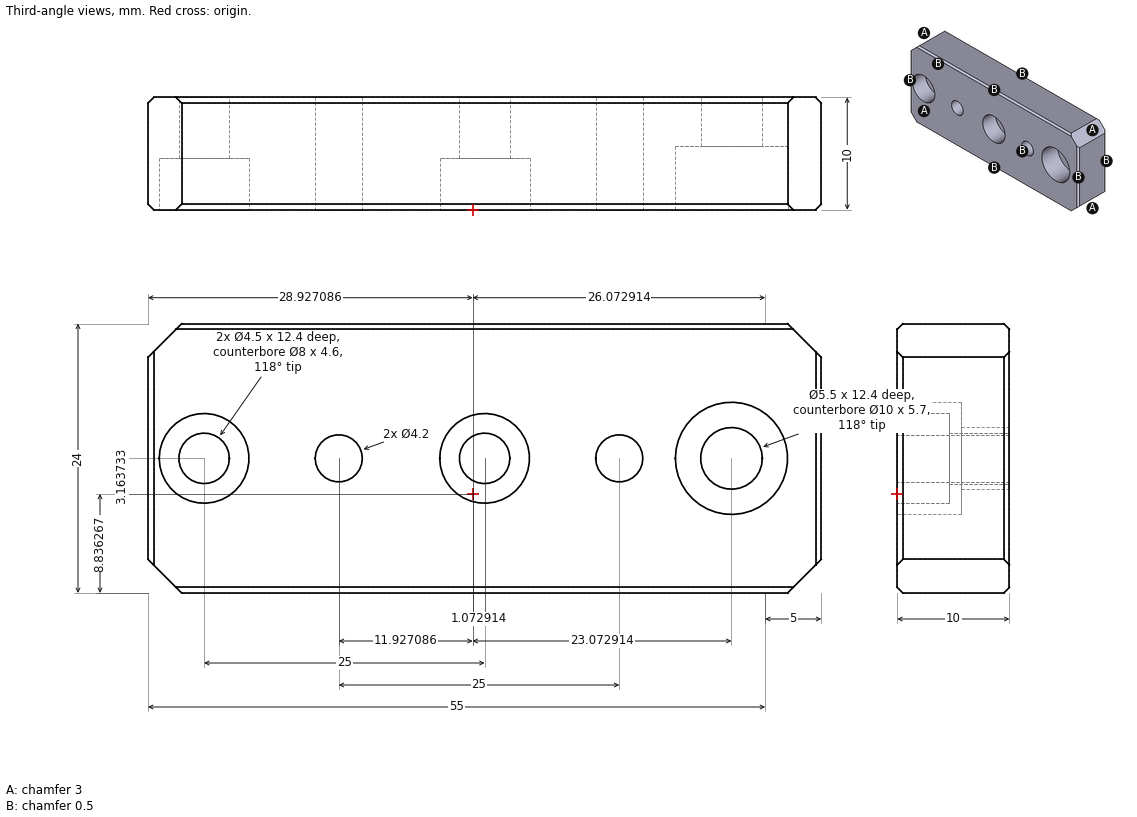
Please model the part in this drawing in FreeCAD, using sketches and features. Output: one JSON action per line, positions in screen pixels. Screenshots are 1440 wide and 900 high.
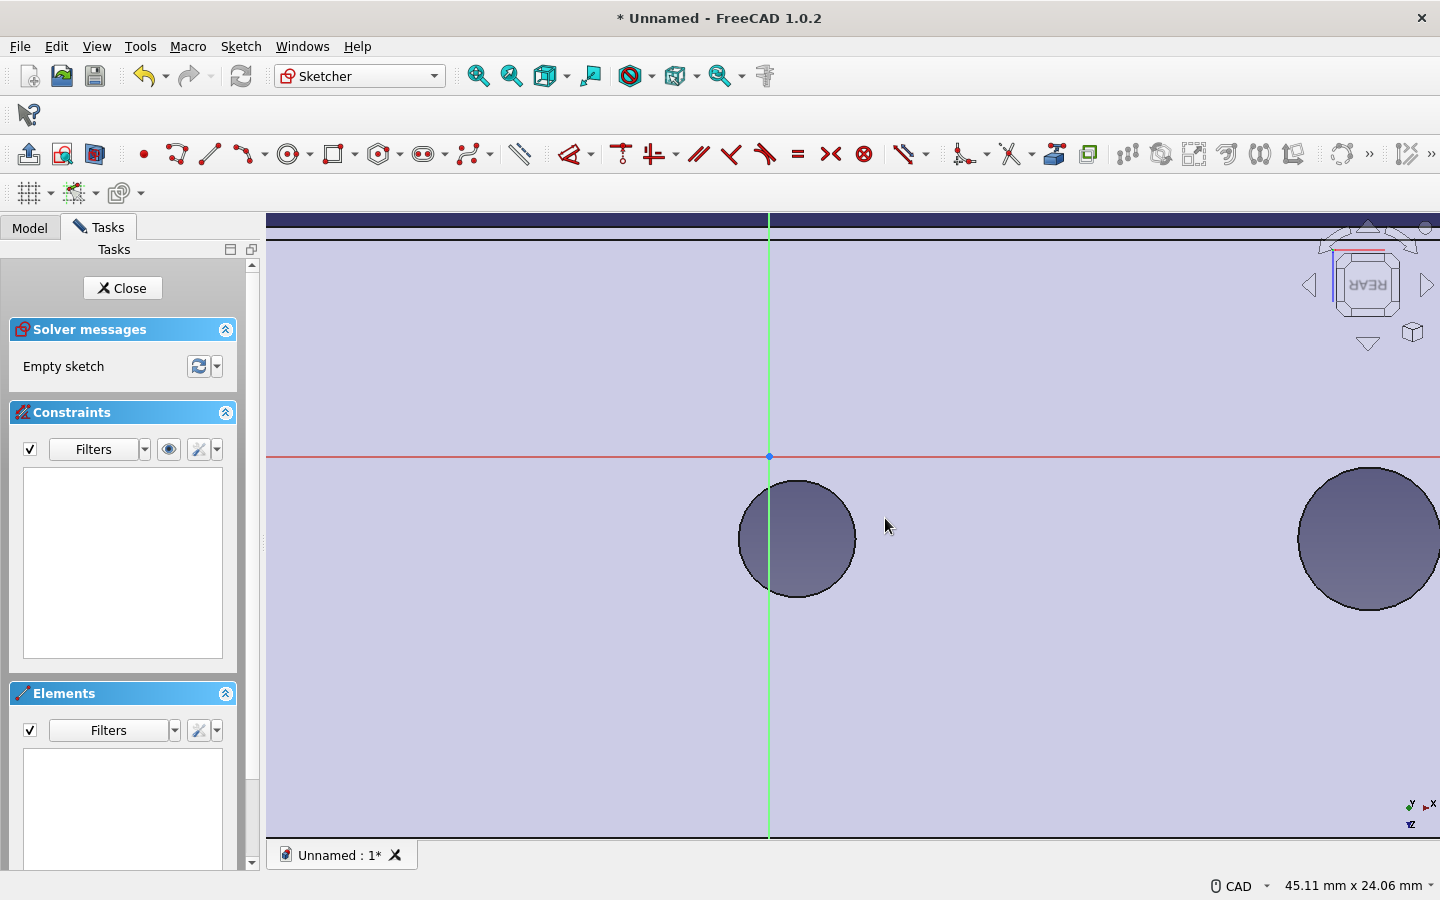
{"action": "key", "text": "g c"}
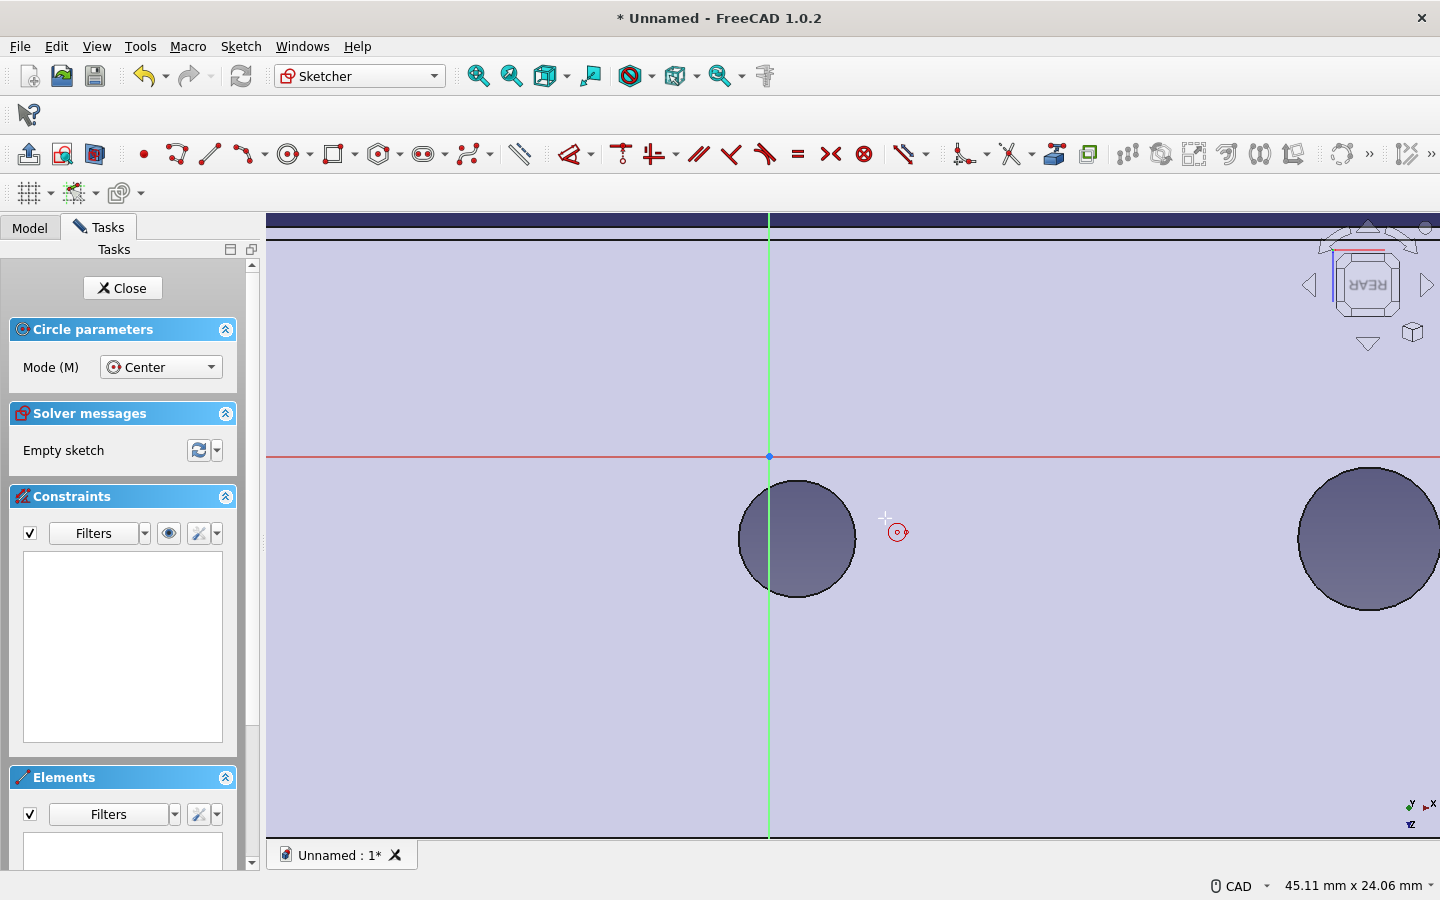
{"action": "left_click", "coordinate": [459, 539]}
{"action": "left_click", "coordinate": [497, 500]}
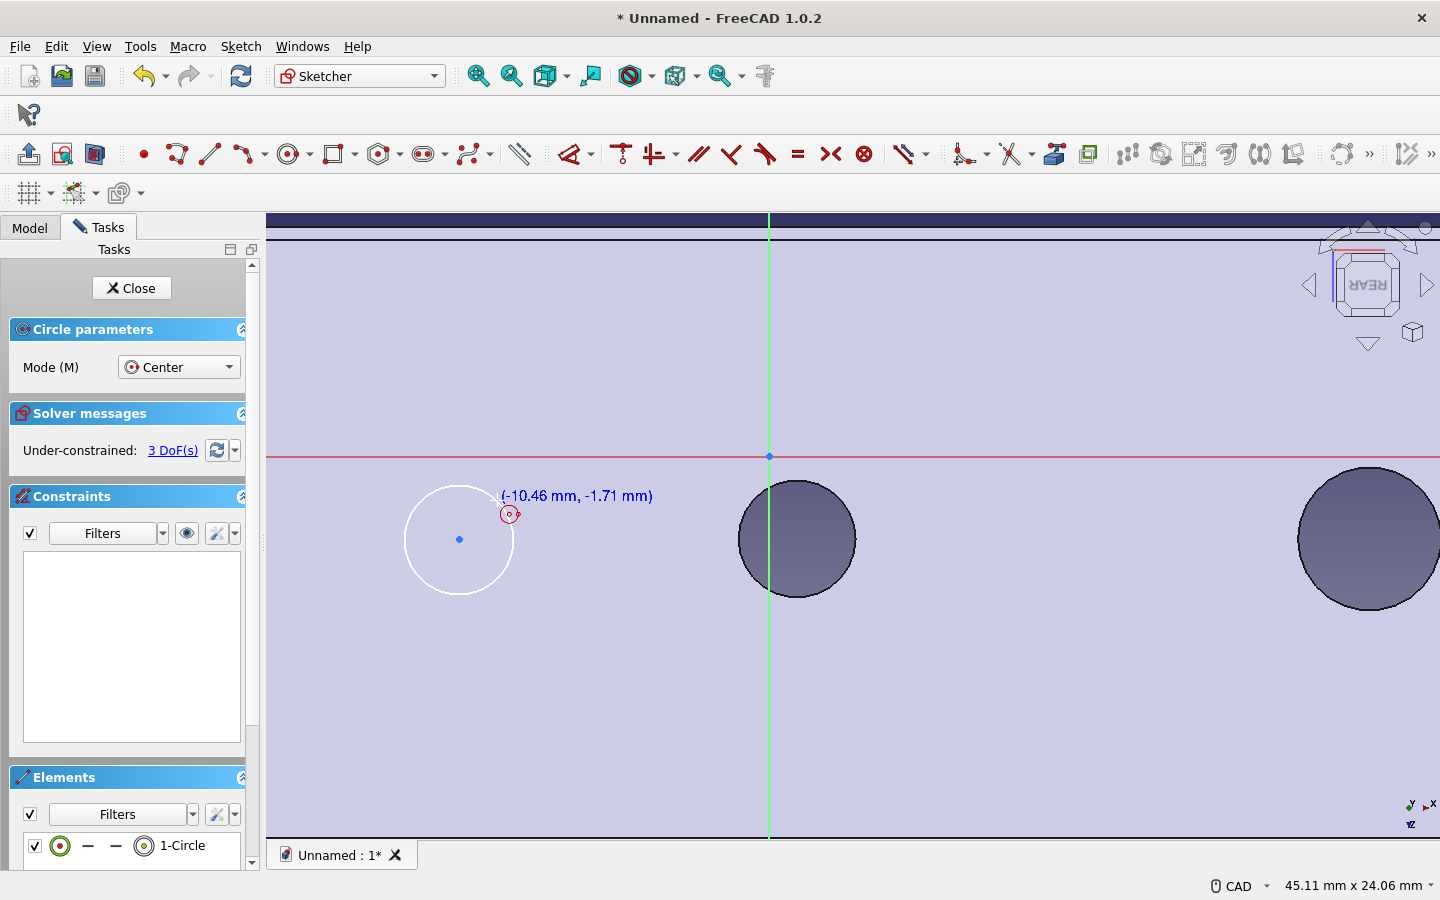
{"action": "left_click", "coordinate": [1109, 539]}
{"action": "left_click", "coordinate": [1148, 500]}
{"action": "key", "text": "Escape"}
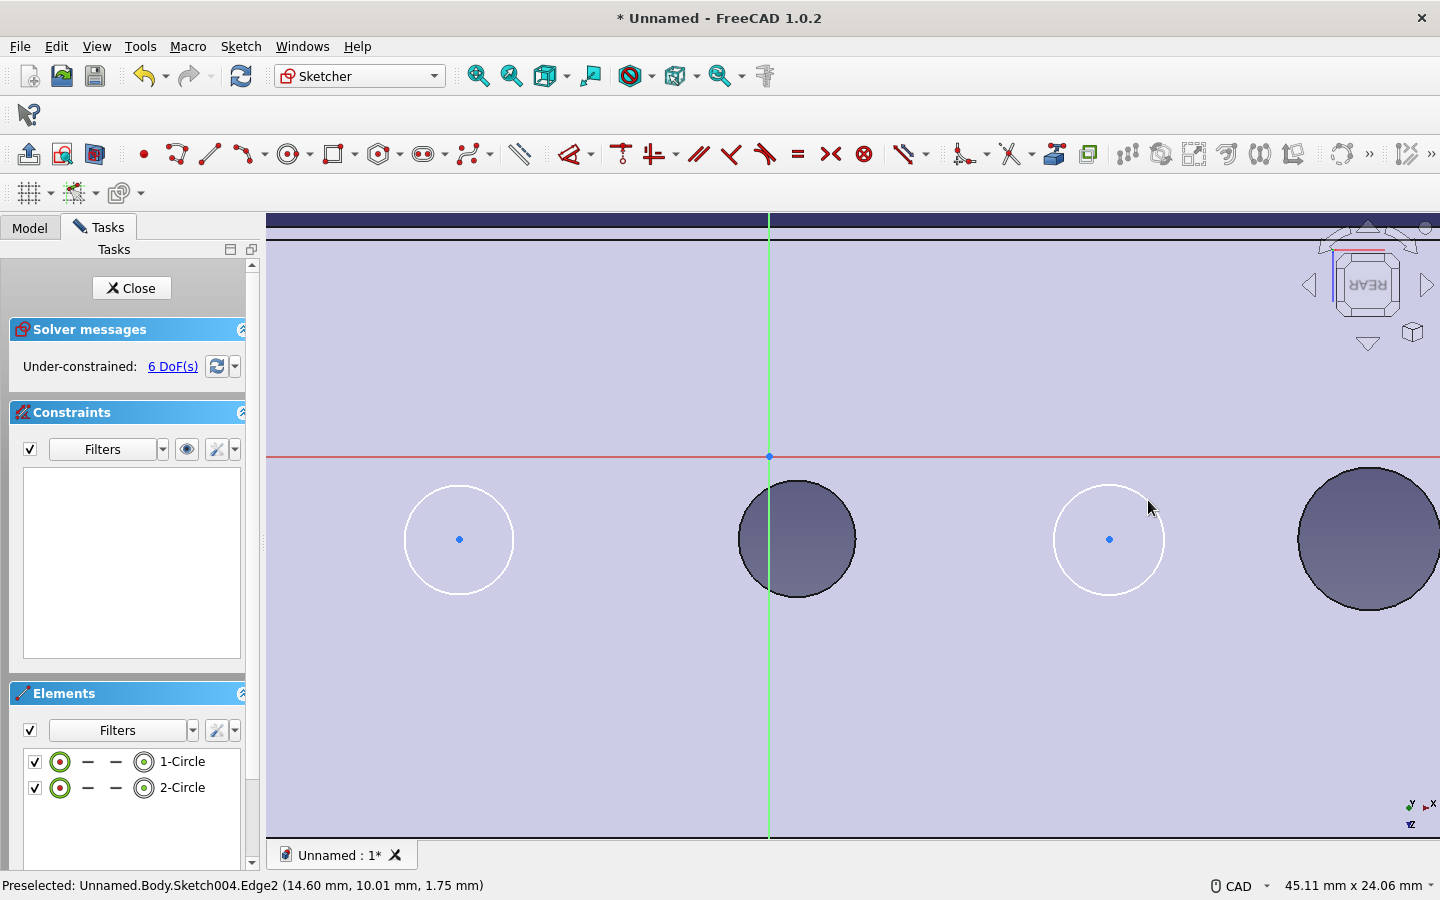
{"action": "left_click", "coordinate": [497, 501]}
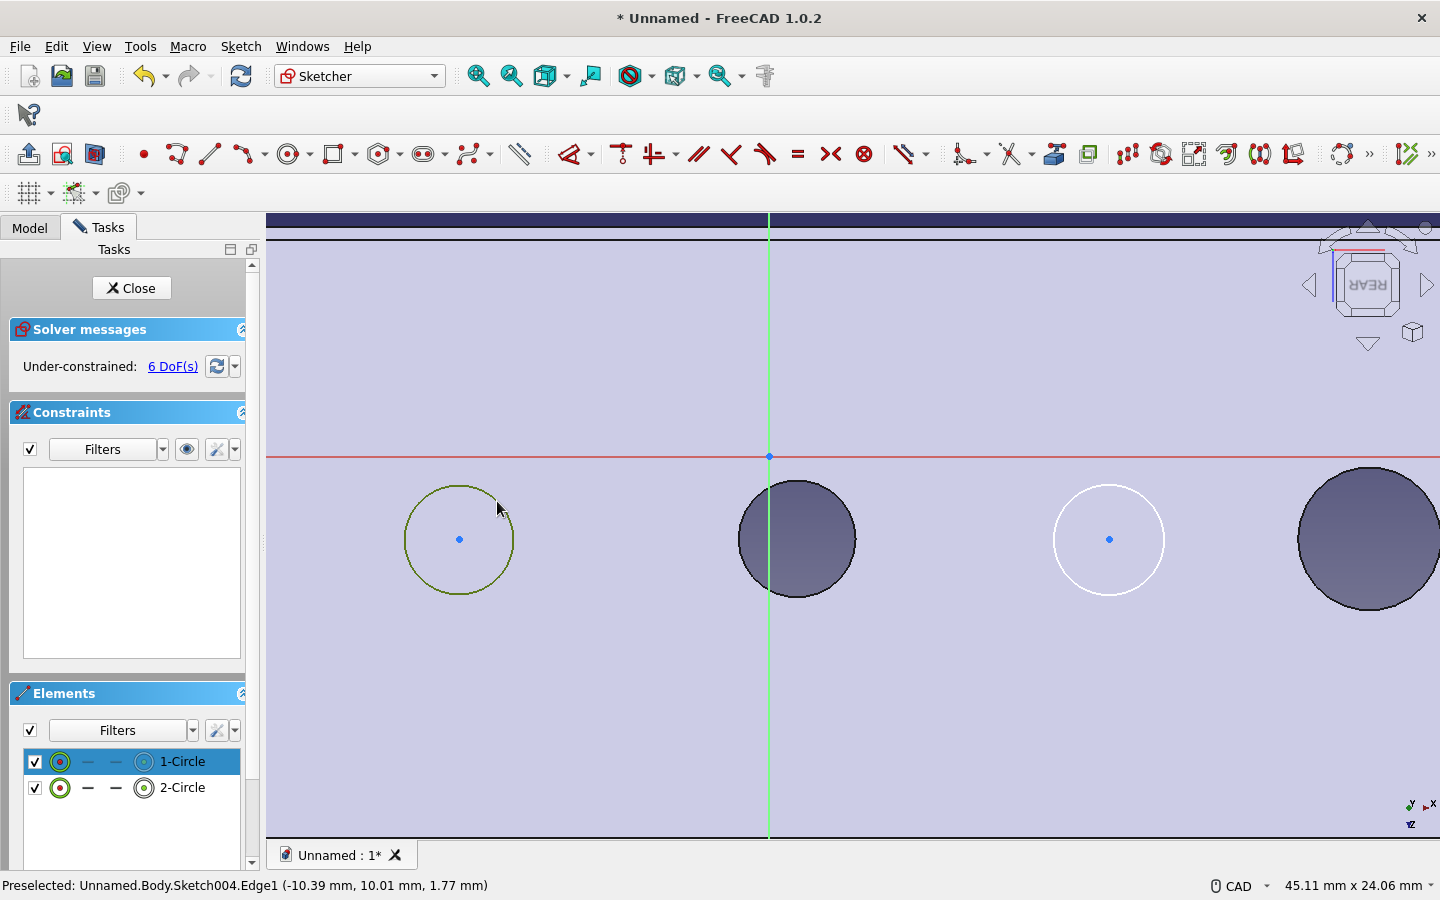
{"action": "left_click", "coordinate": [1148, 501]}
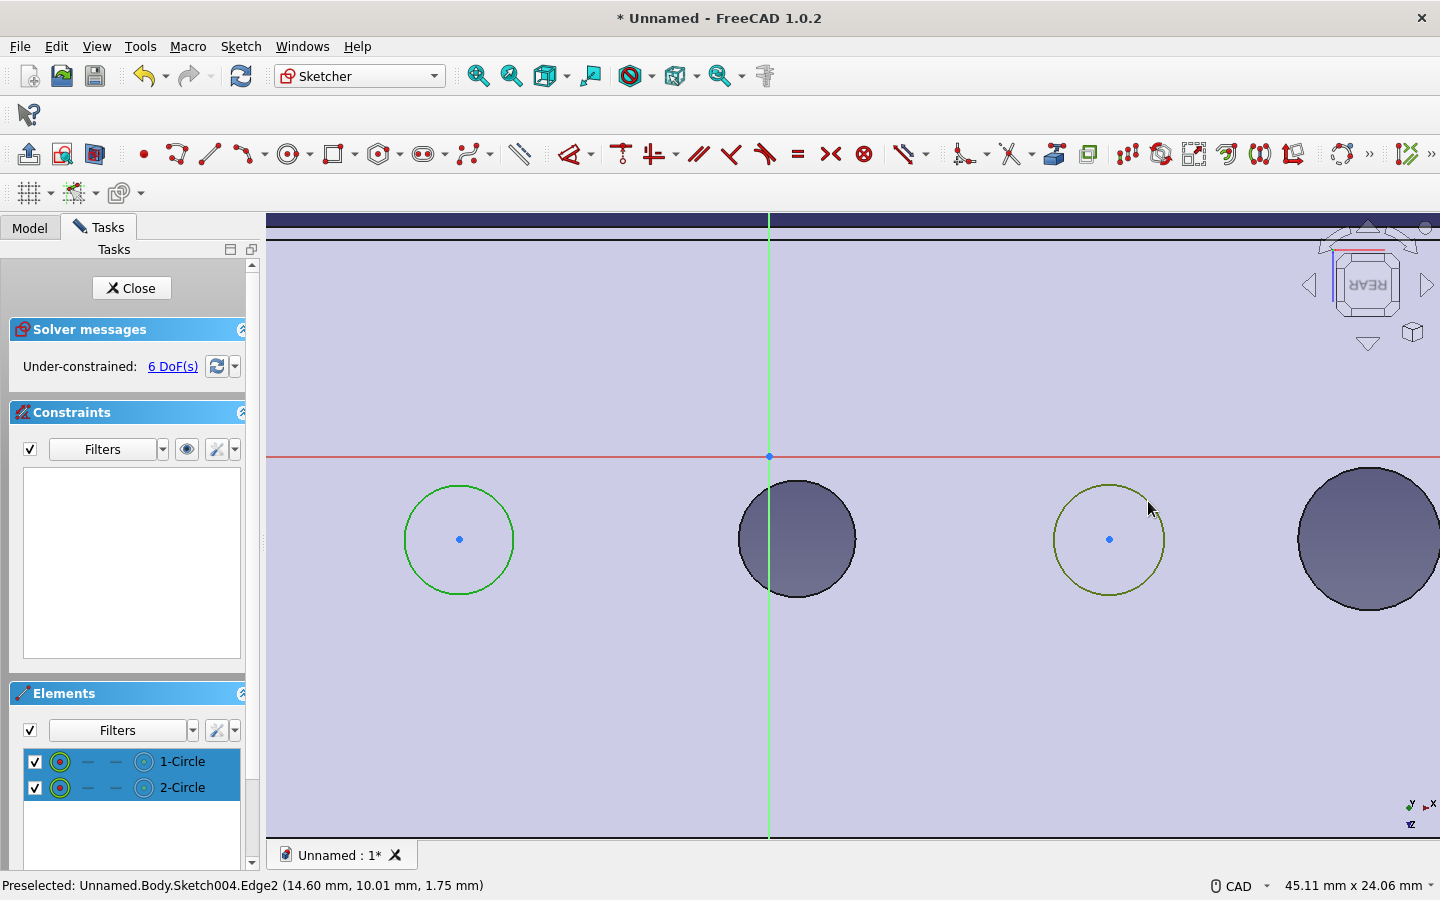
{"action": "key", "text": "e"}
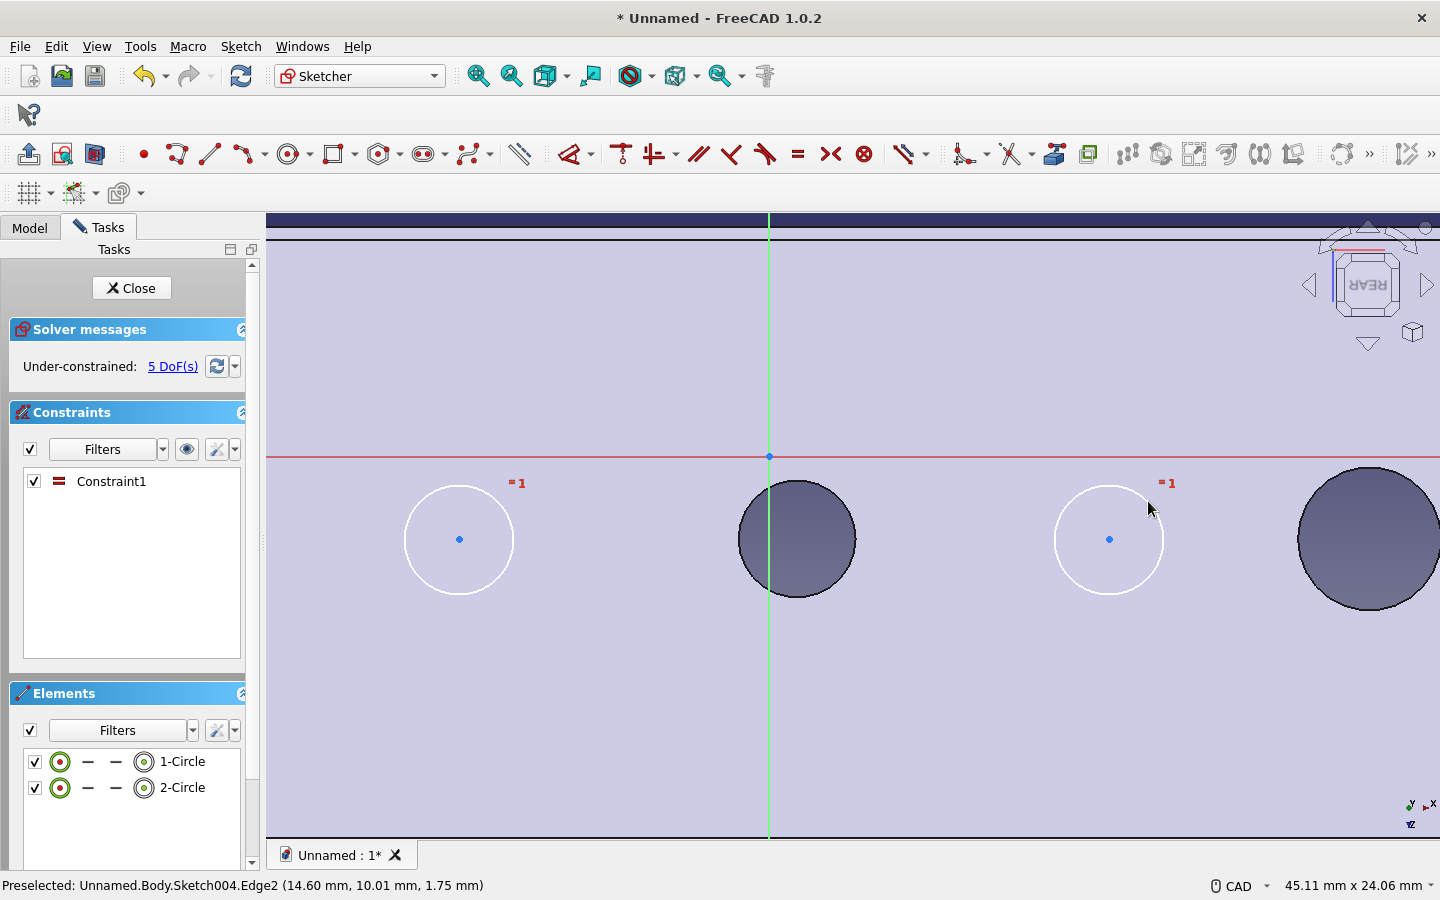
{"action": "left_click", "coordinate": [459, 540]}